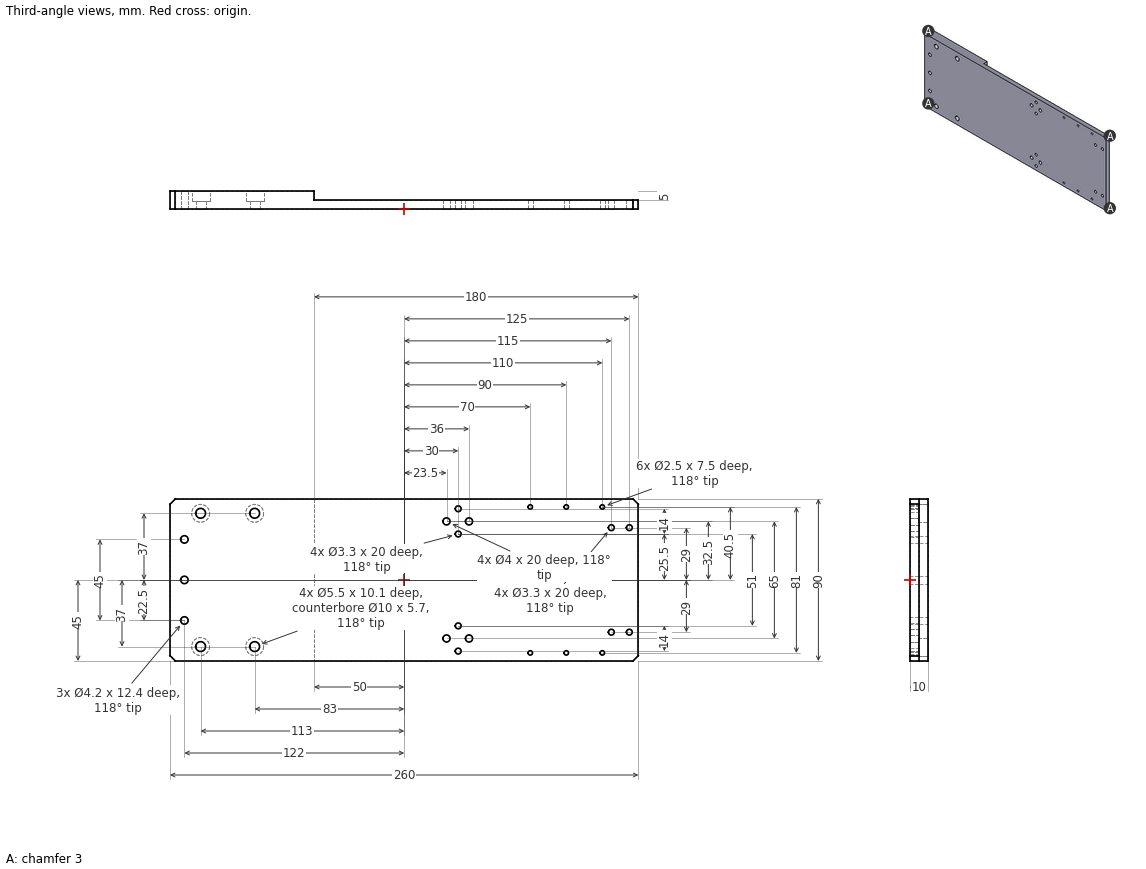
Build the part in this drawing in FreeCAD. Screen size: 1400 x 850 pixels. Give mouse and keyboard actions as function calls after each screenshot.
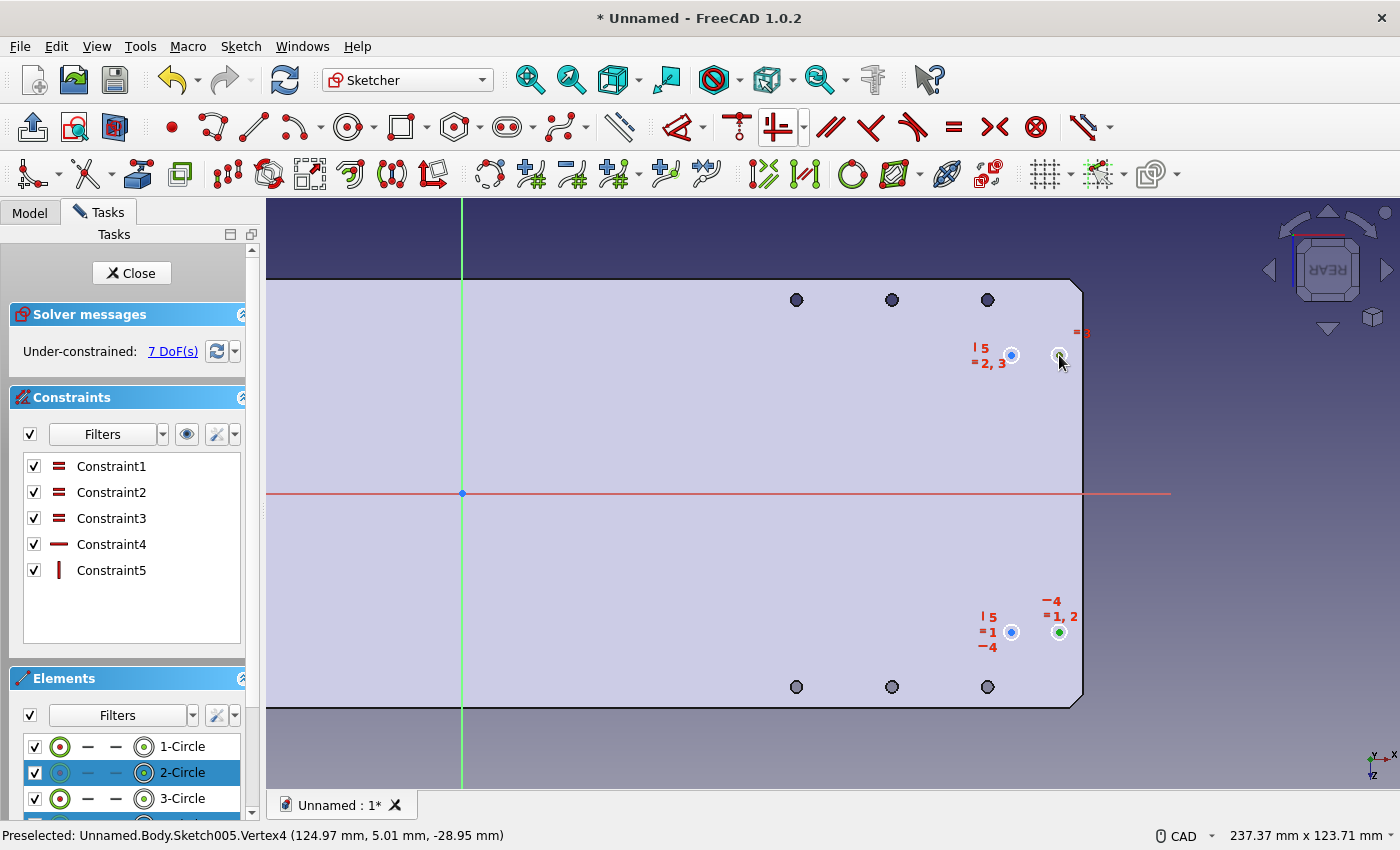
key(v)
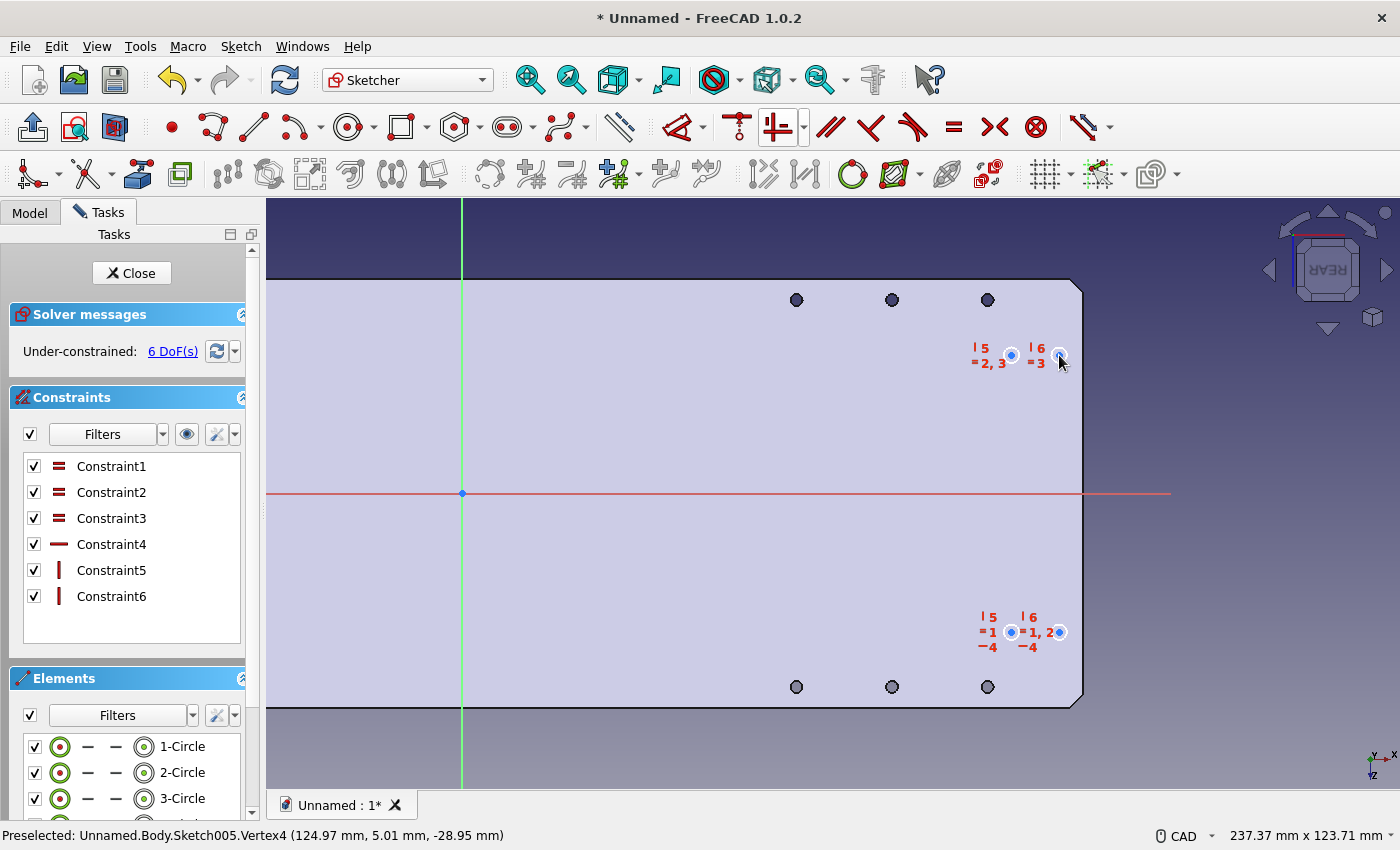
click(1012, 355)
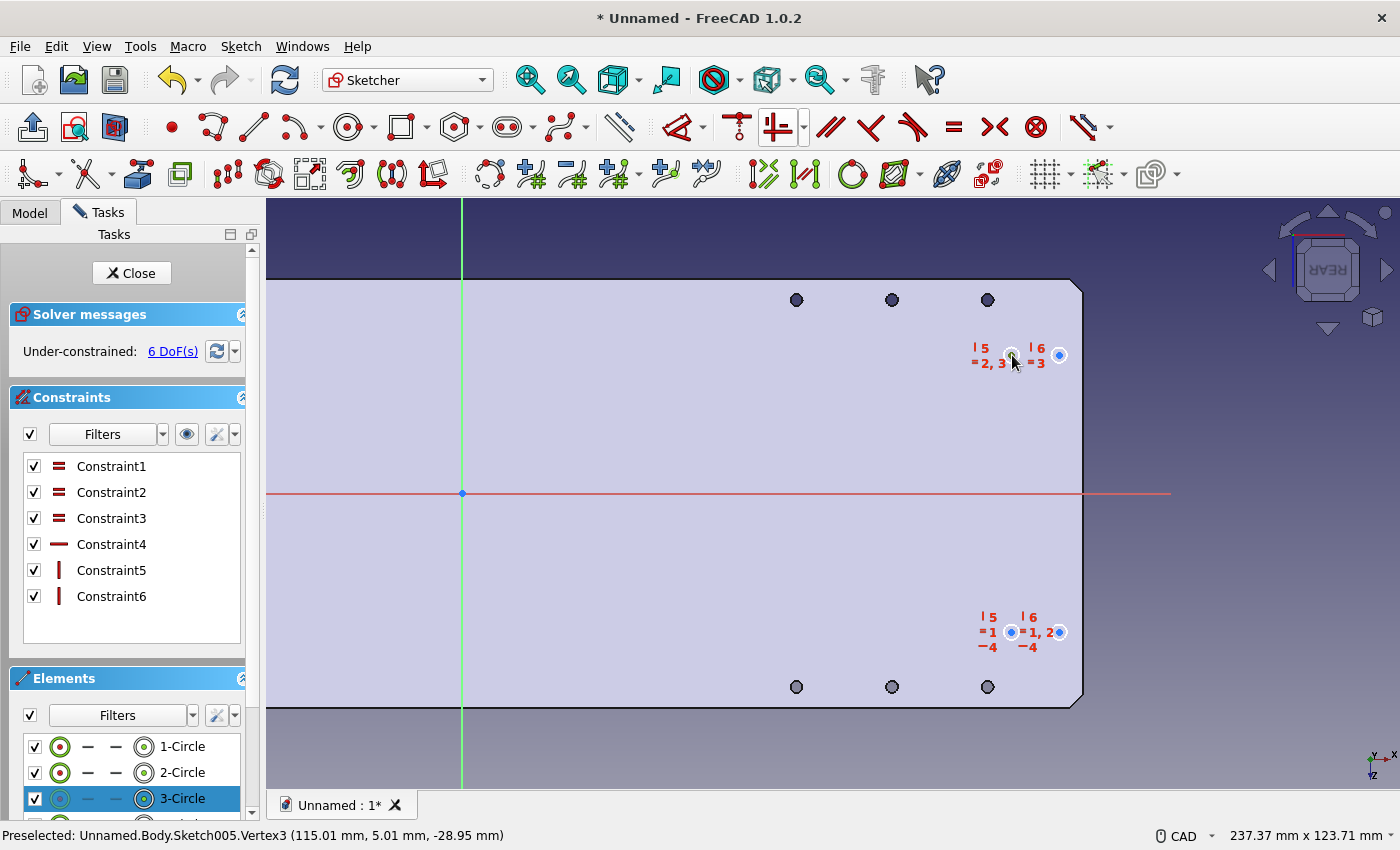
click(1059, 355)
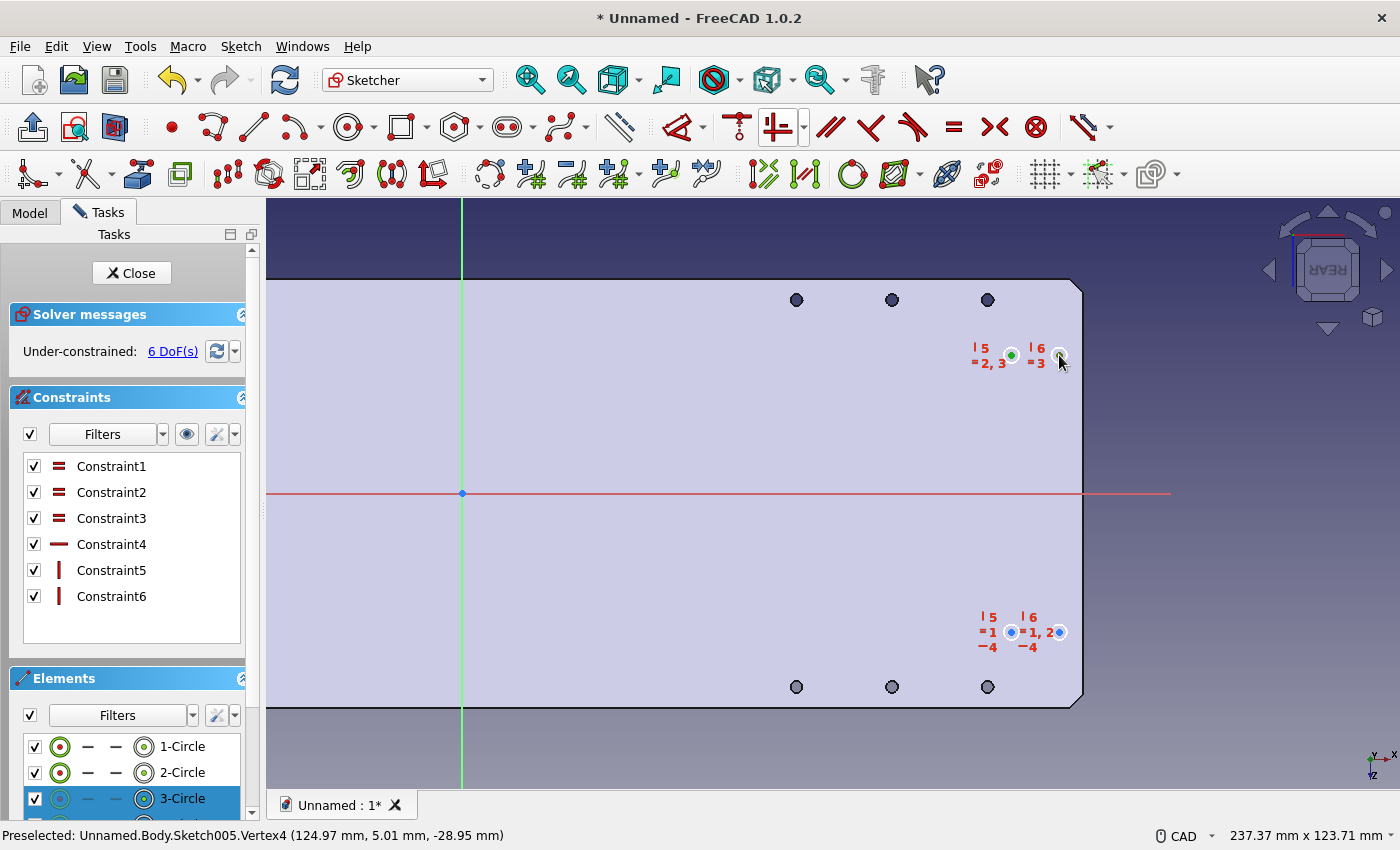
click(804, 128)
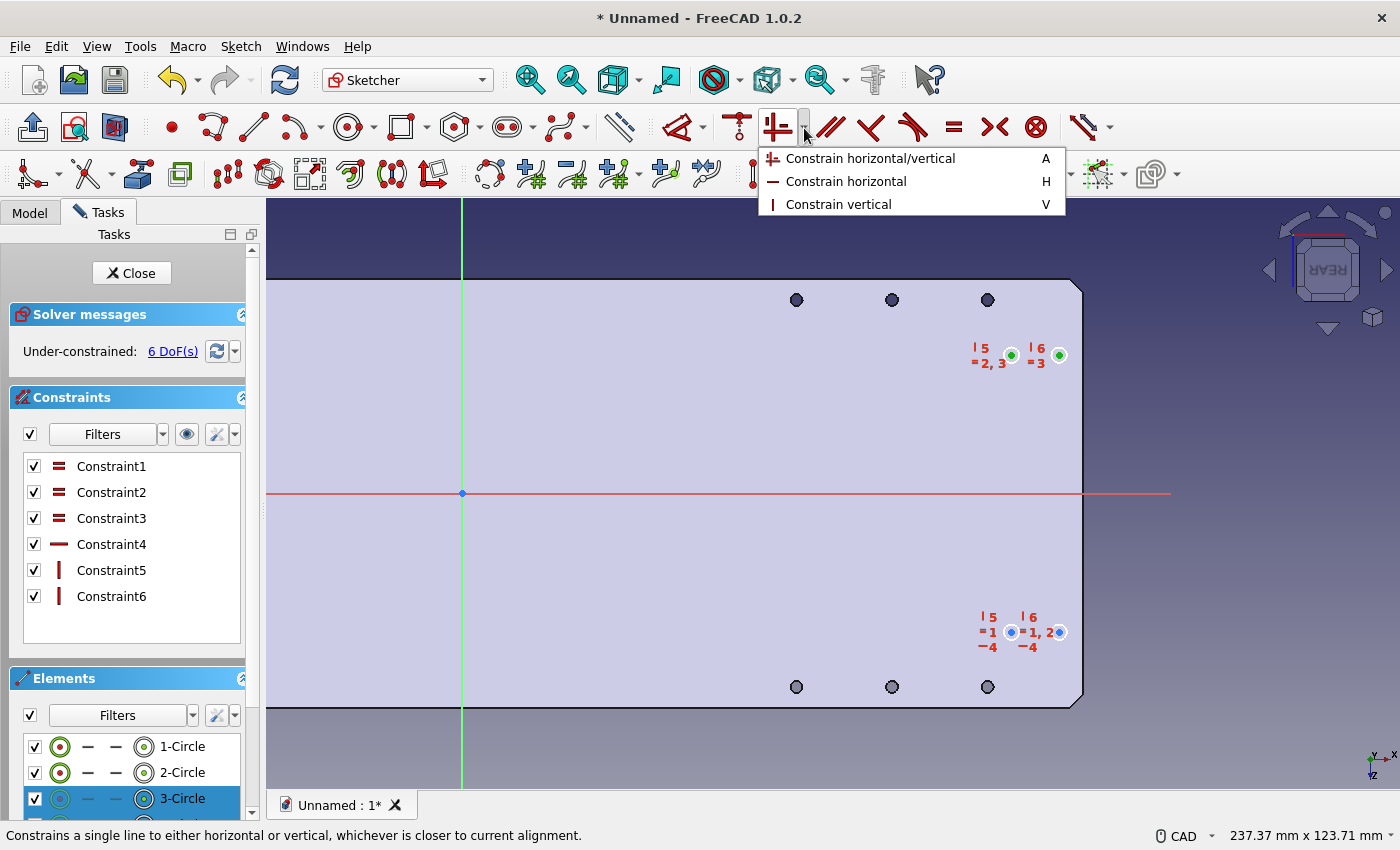
click(912, 182)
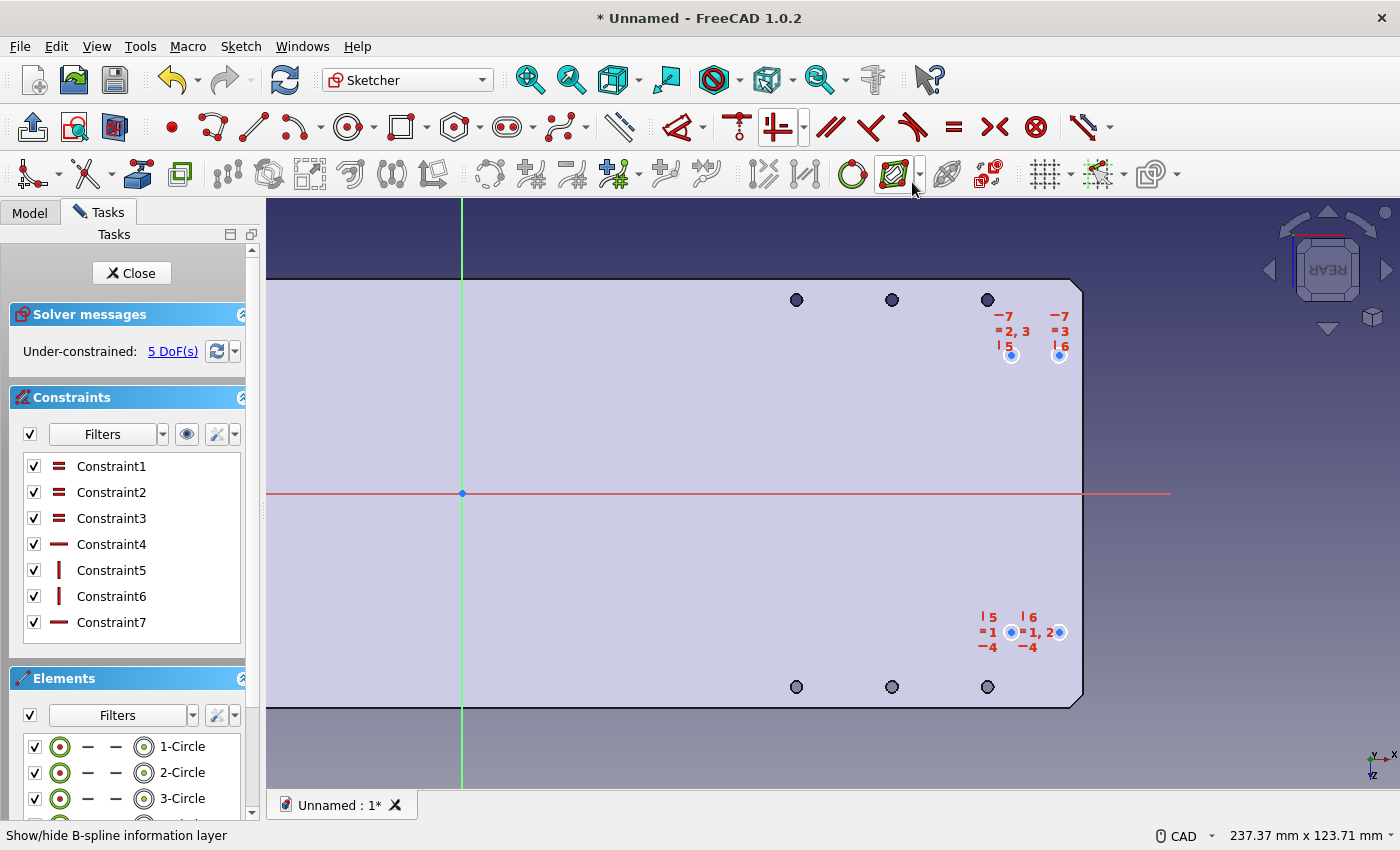
click(676, 128)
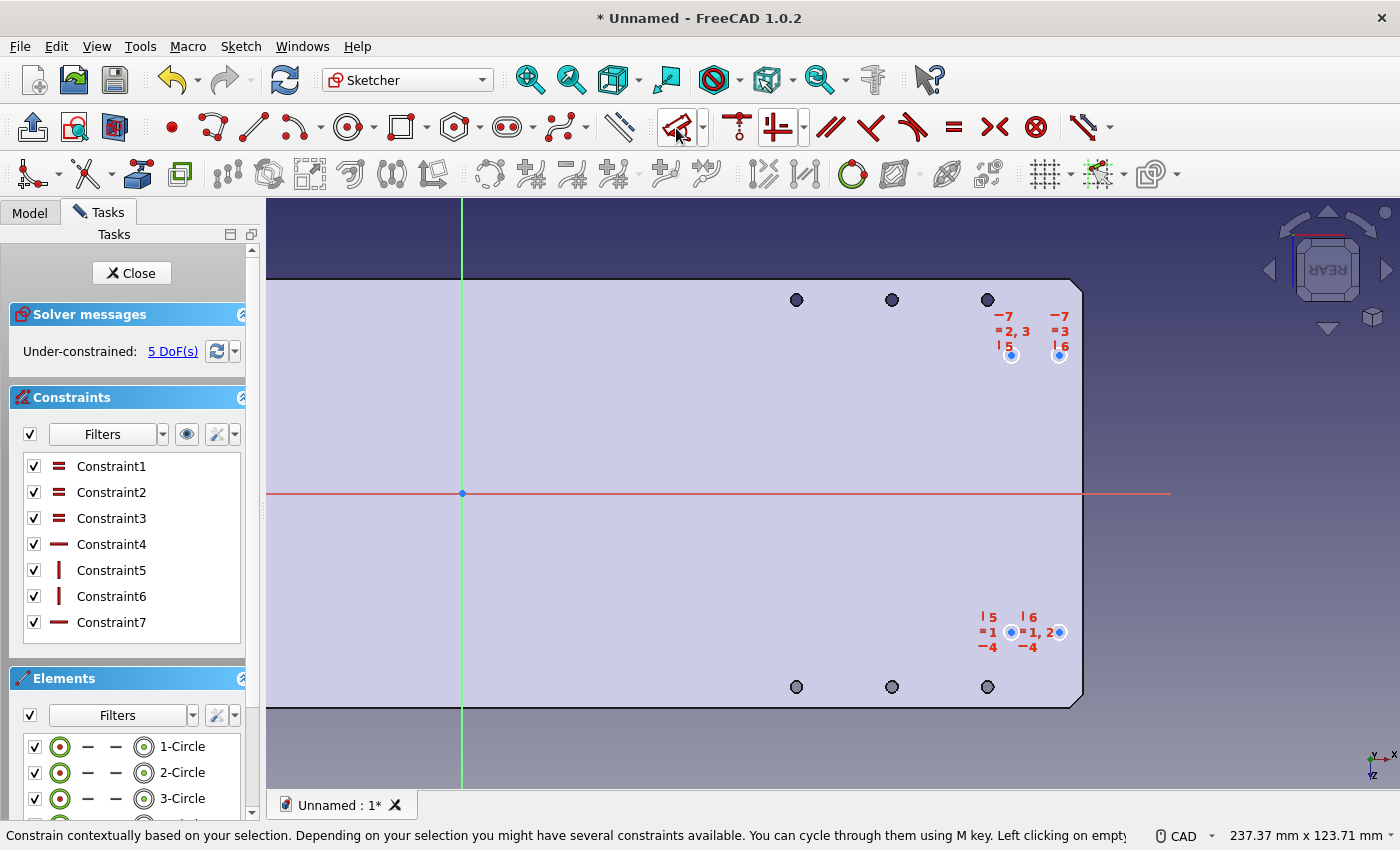
scroll(1006, 638, up, 5)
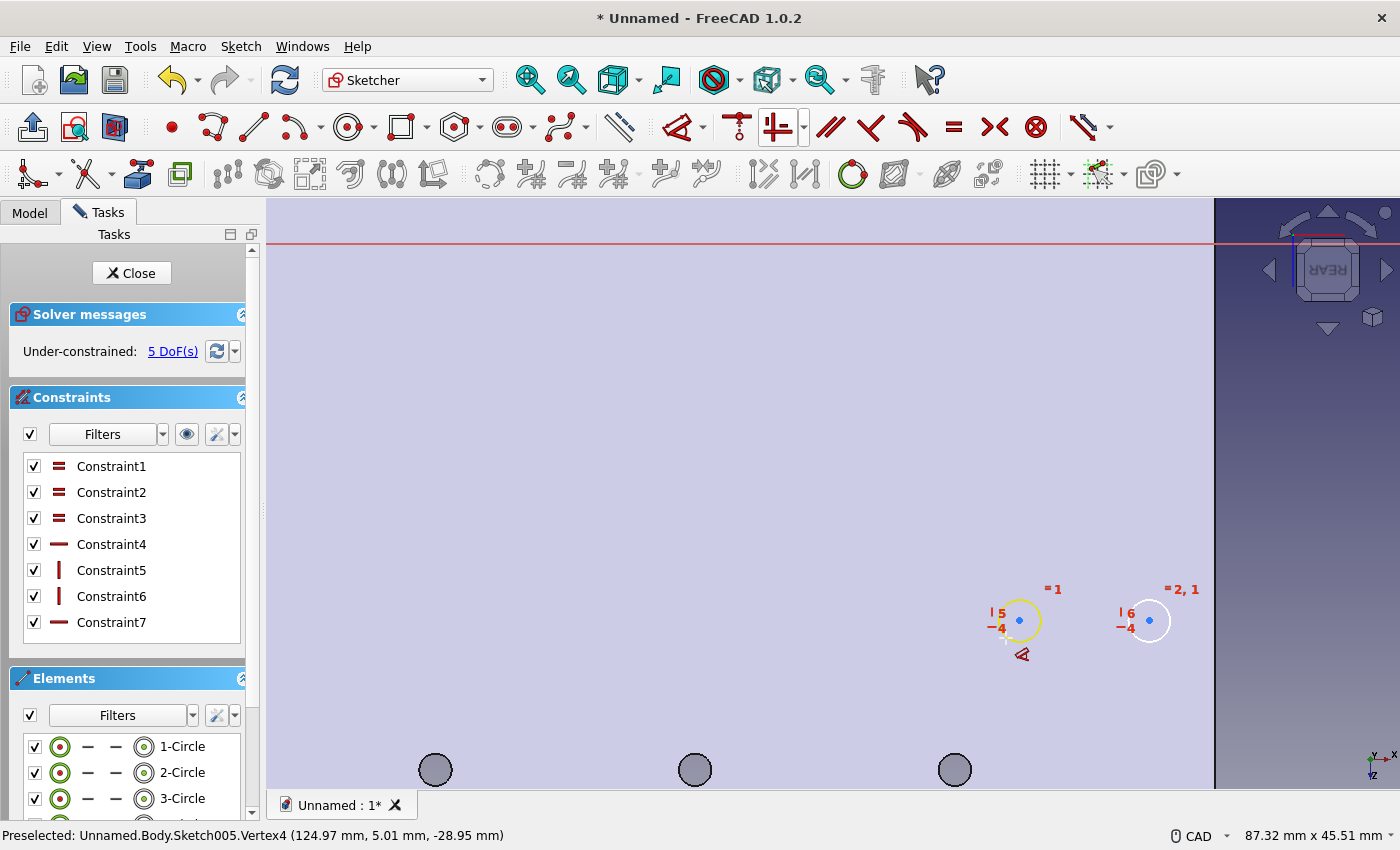
click(1005, 636)
click(982, 659)